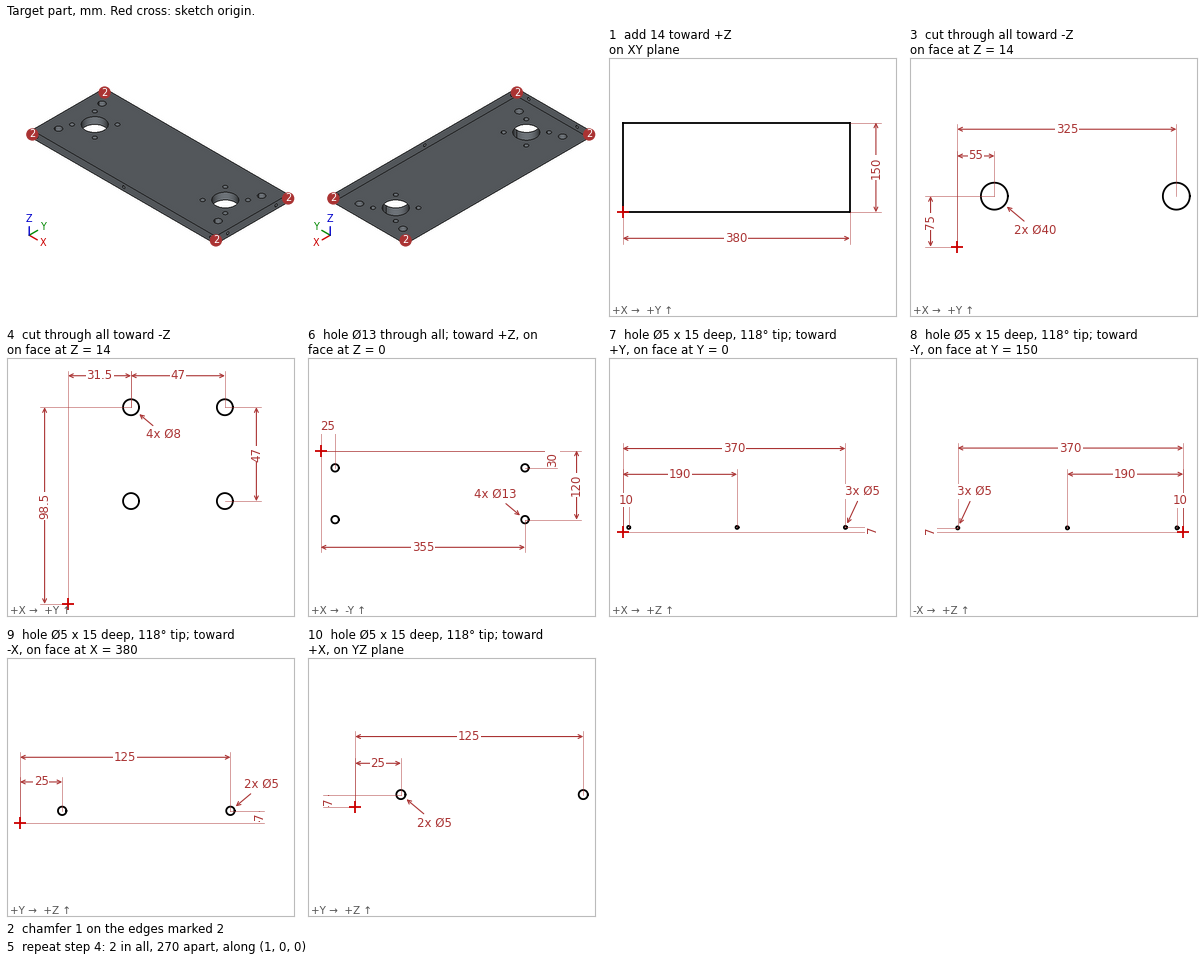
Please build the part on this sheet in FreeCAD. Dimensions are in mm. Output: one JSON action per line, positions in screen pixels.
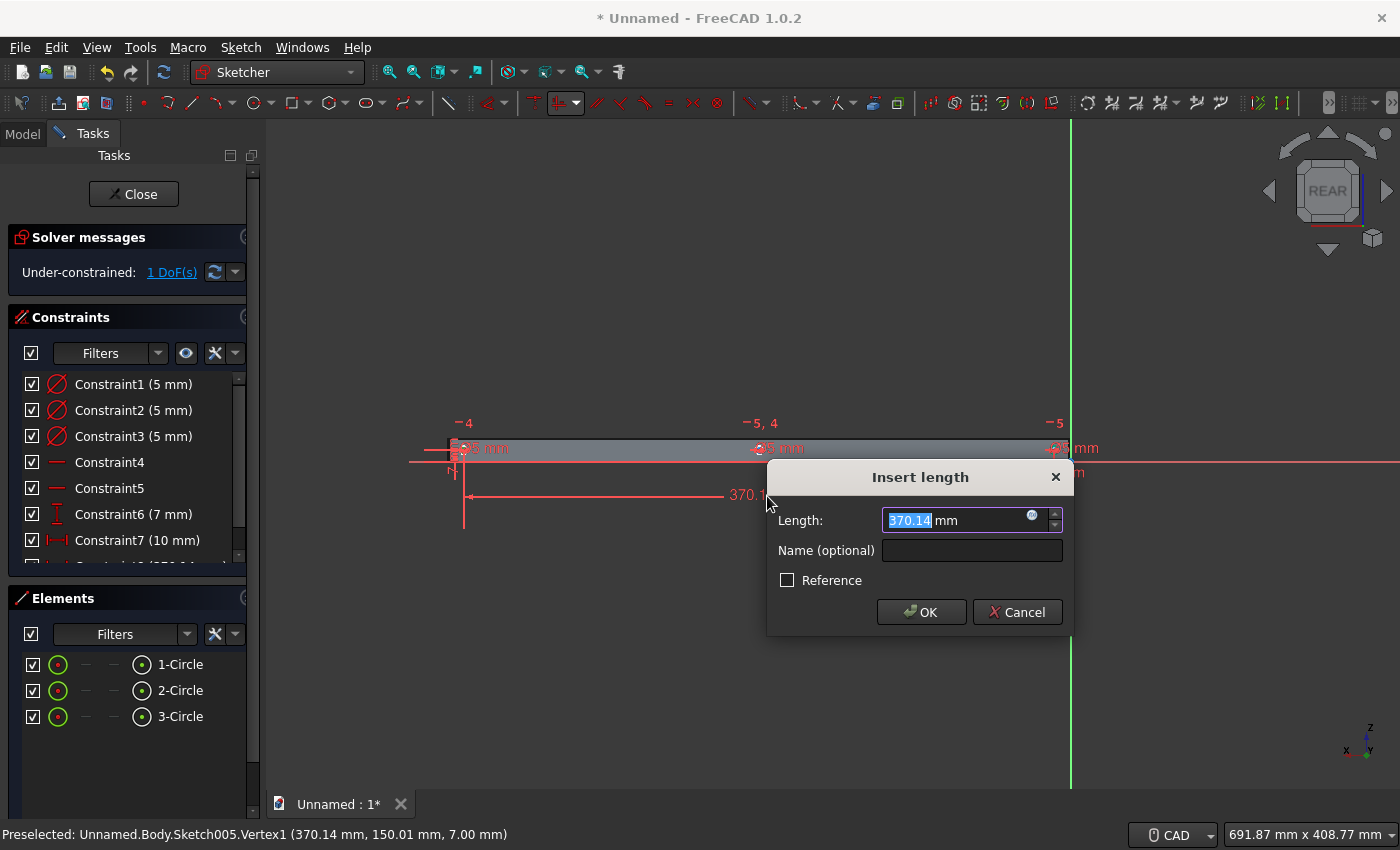
{"action": "type", "text": "370"}
{"action": "key", "text": "Return"}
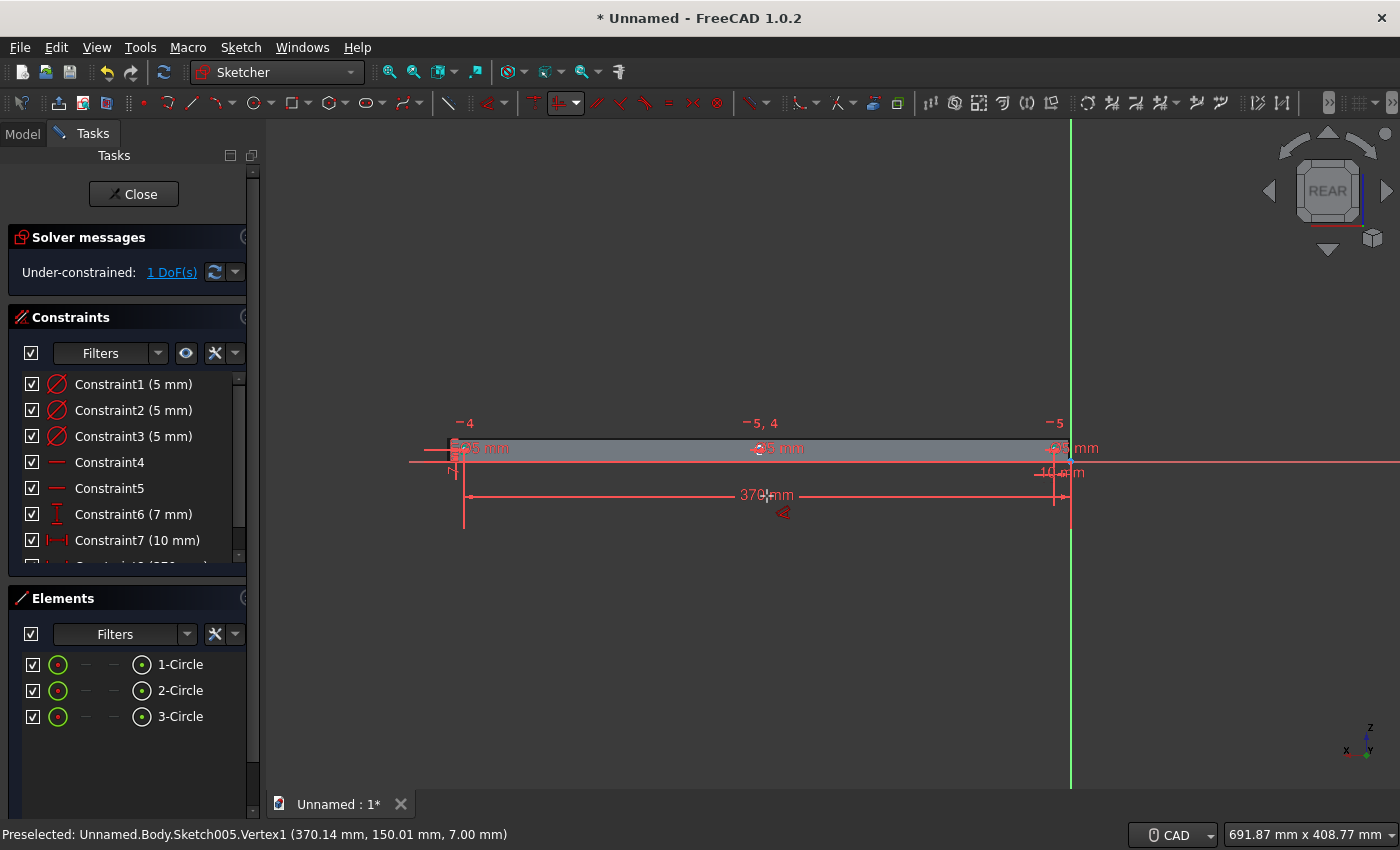
{"action": "left_click", "coordinate": [759, 450]}
{"action": "left_click", "coordinate": [915, 496]}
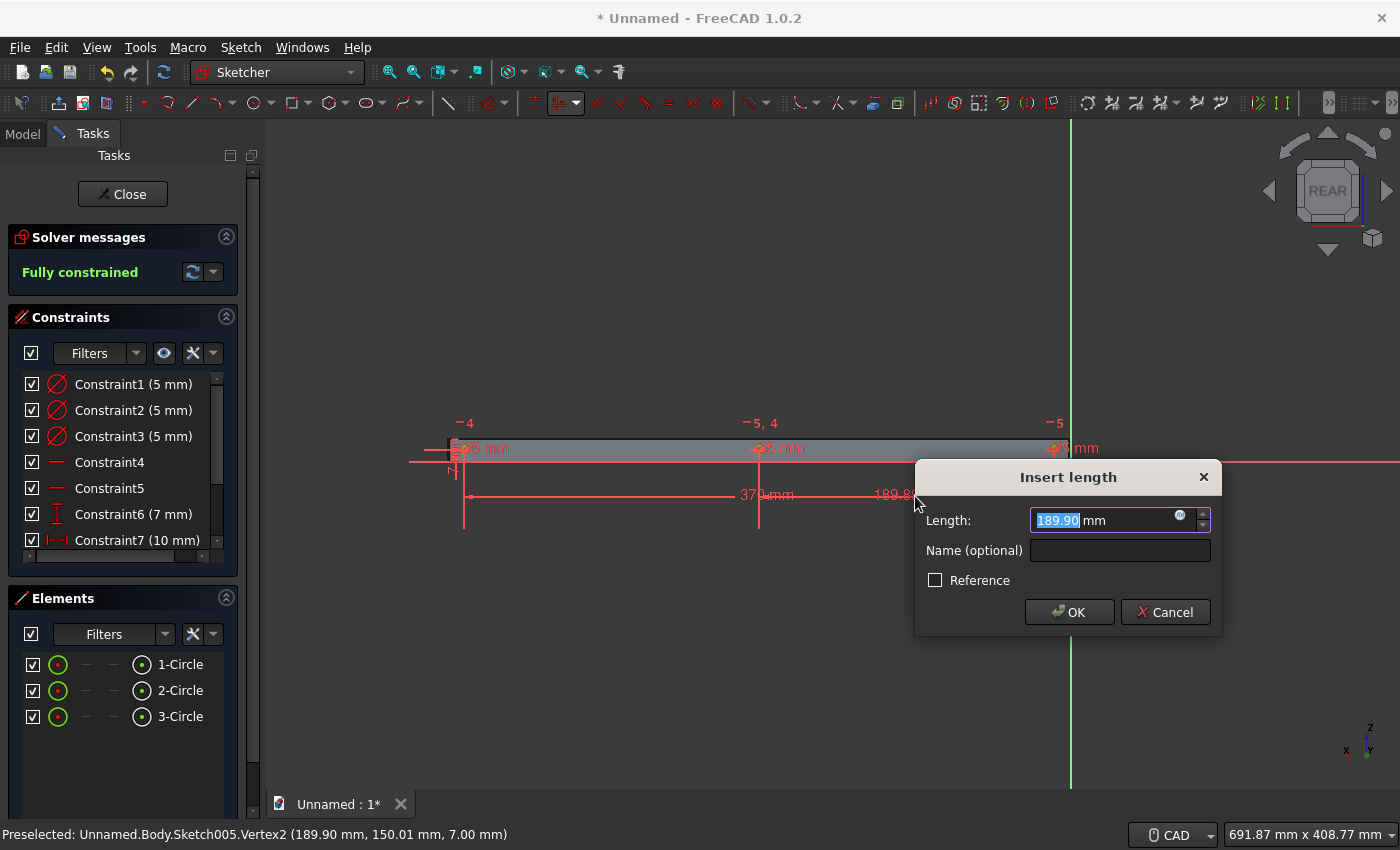
{"action": "type", "text": "190"}
{"action": "key", "text": "Return"}
{"action": "key", "text": "Escape"}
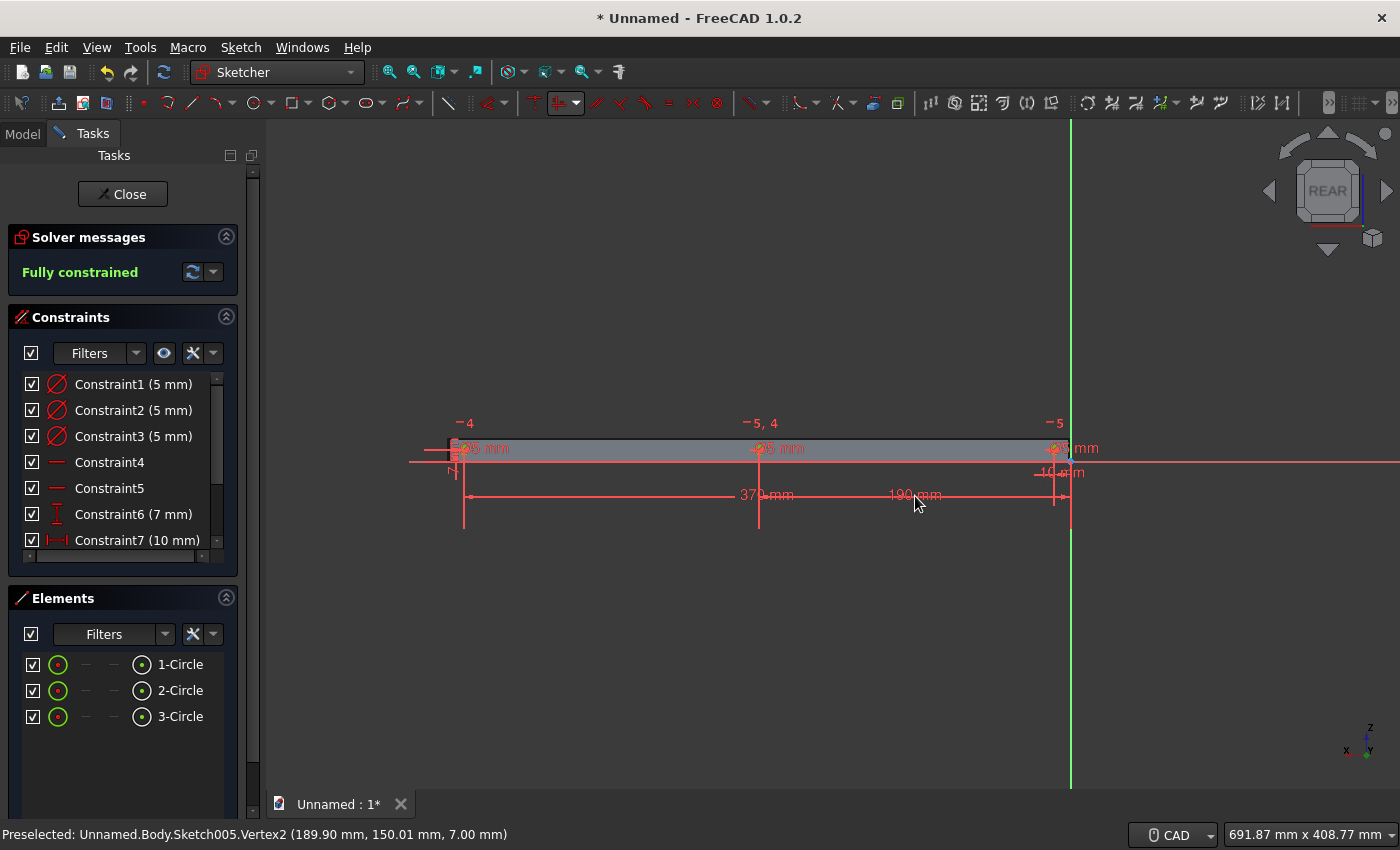
{"action": "left_click", "coordinate": [123, 194]}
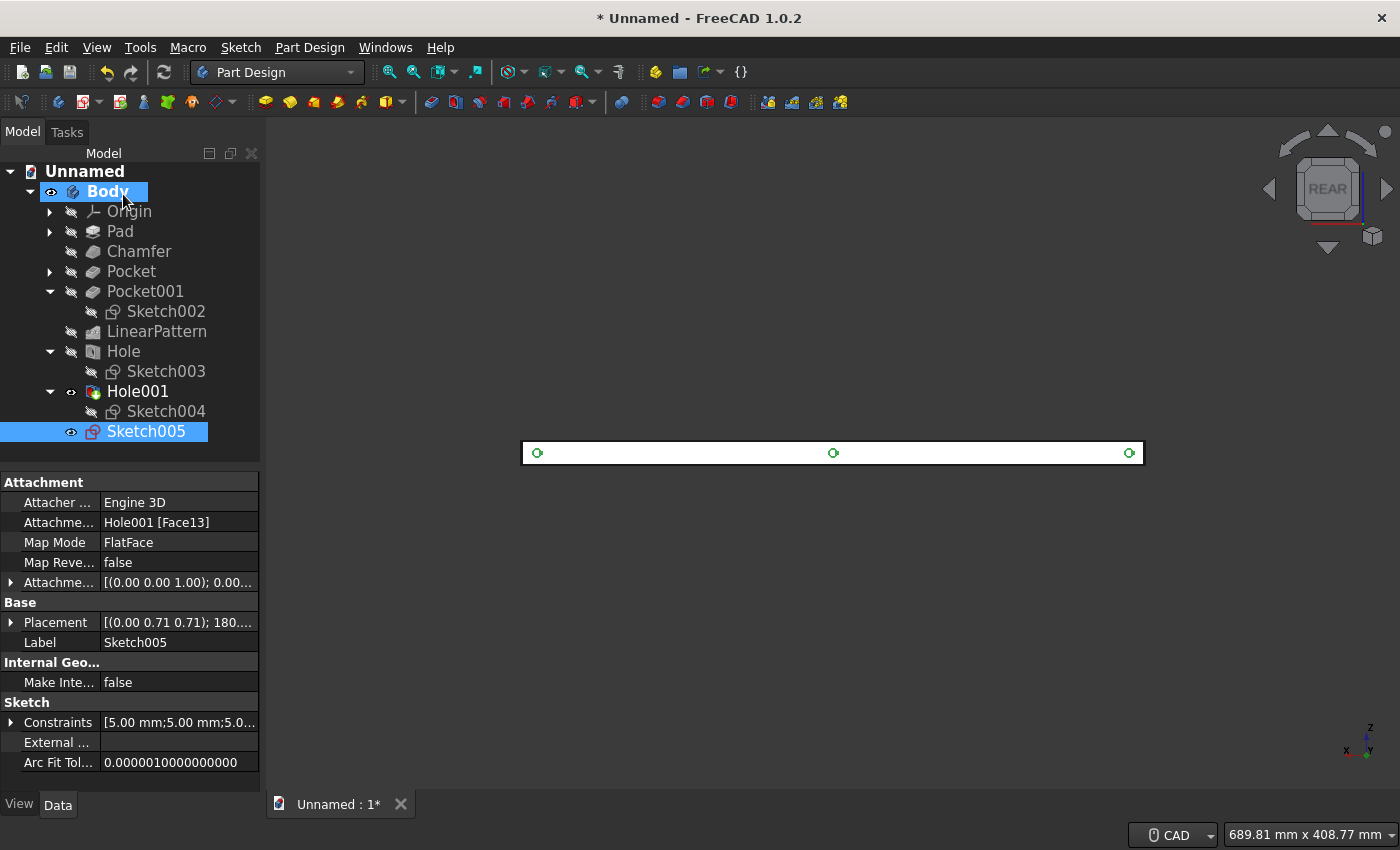
{"action": "left_click", "coordinate": [456, 102]}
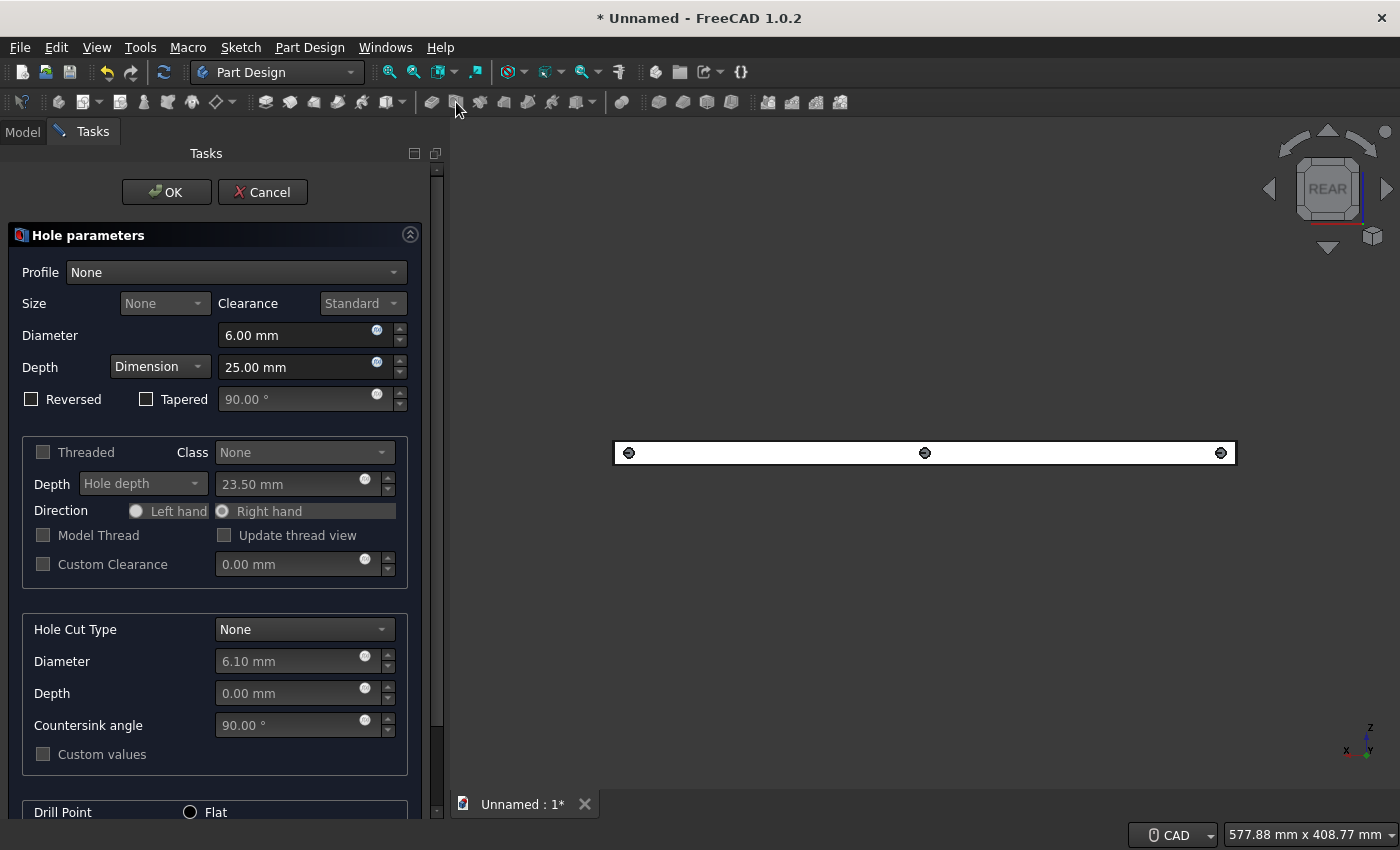
{"action": "triple_click", "coordinate": [305, 335]}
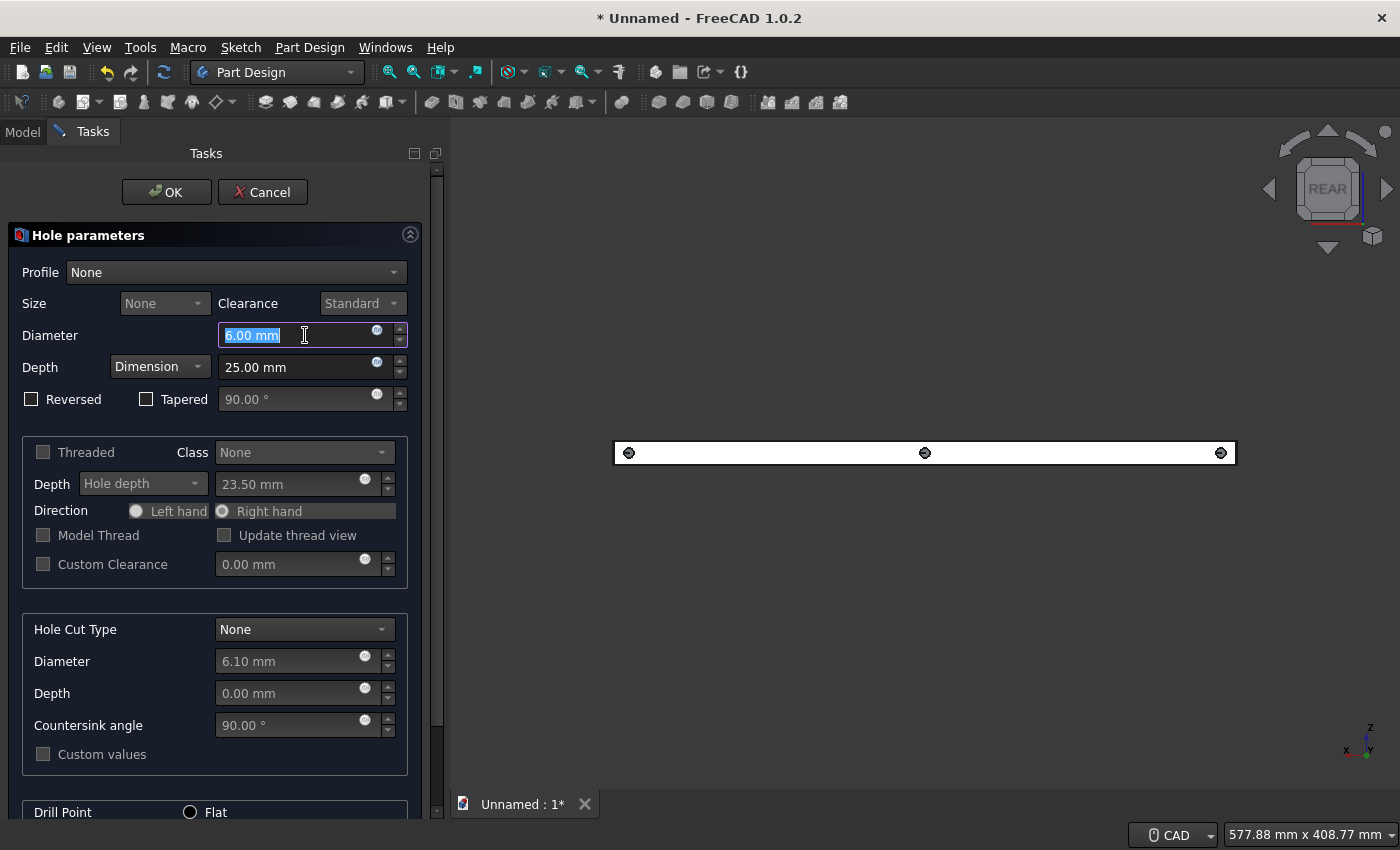
{"action": "type", "text": "5"}
{"action": "key", "text": "Tab"}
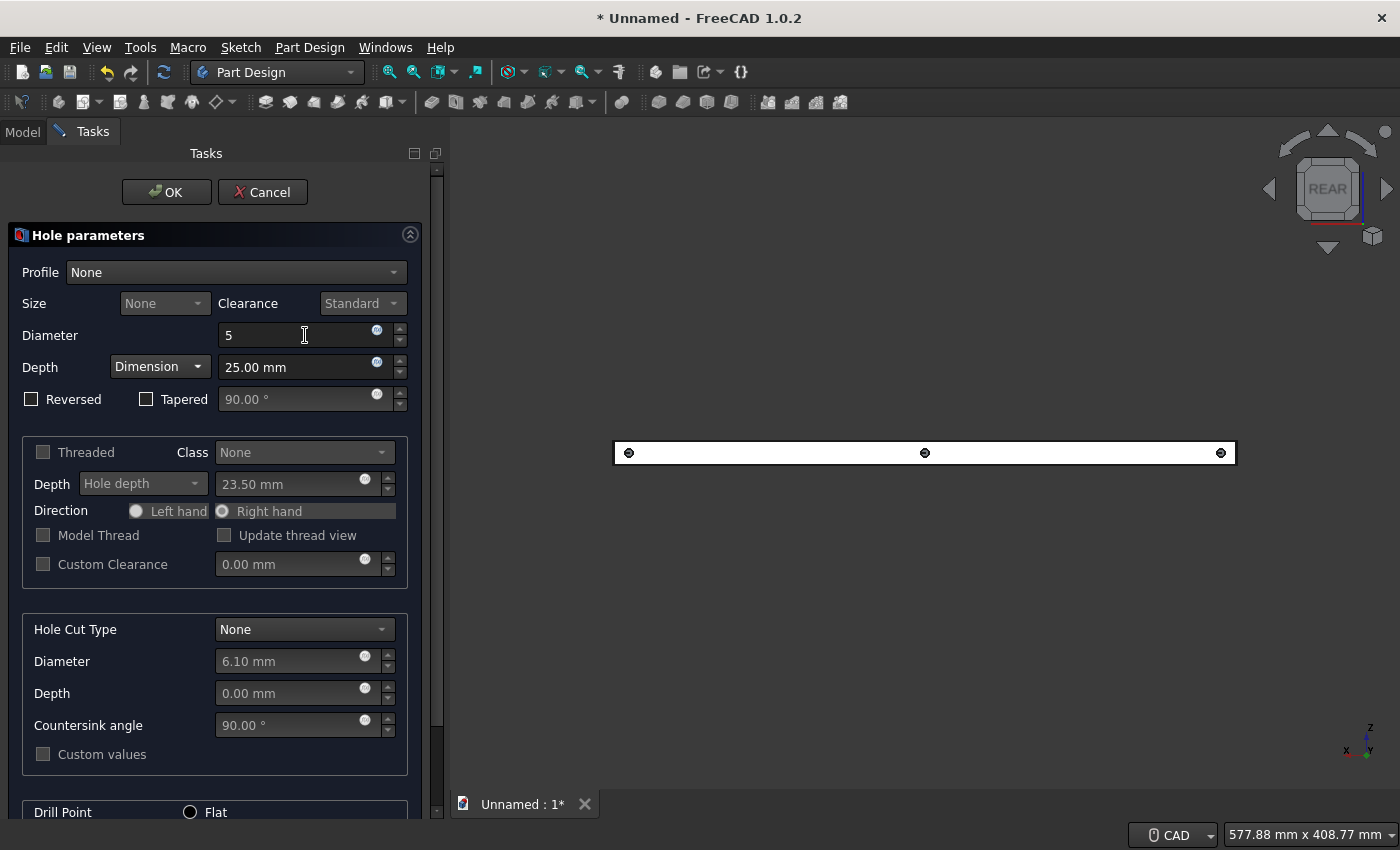
{"action": "triple_click", "coordinate": [305, 367]}